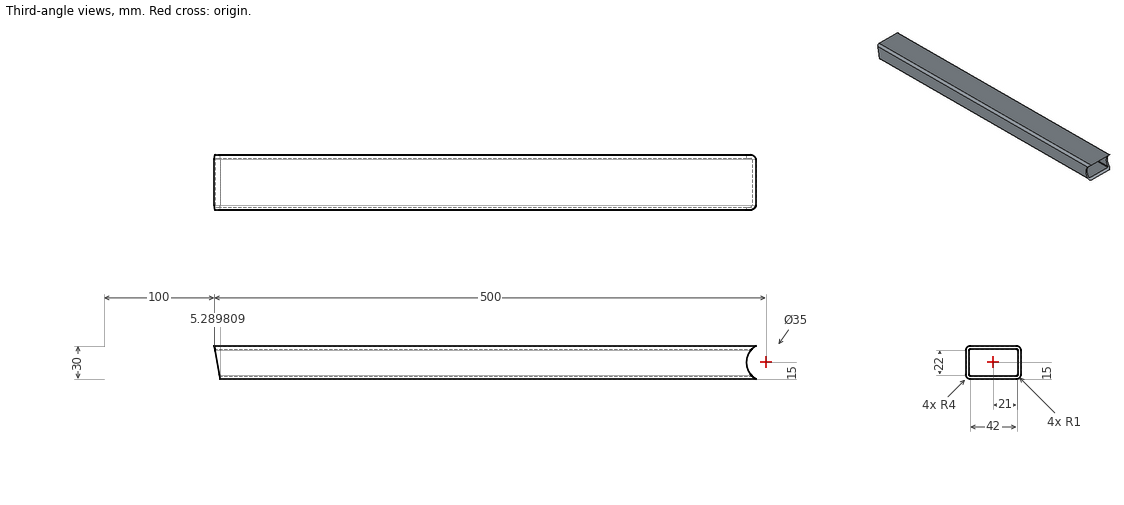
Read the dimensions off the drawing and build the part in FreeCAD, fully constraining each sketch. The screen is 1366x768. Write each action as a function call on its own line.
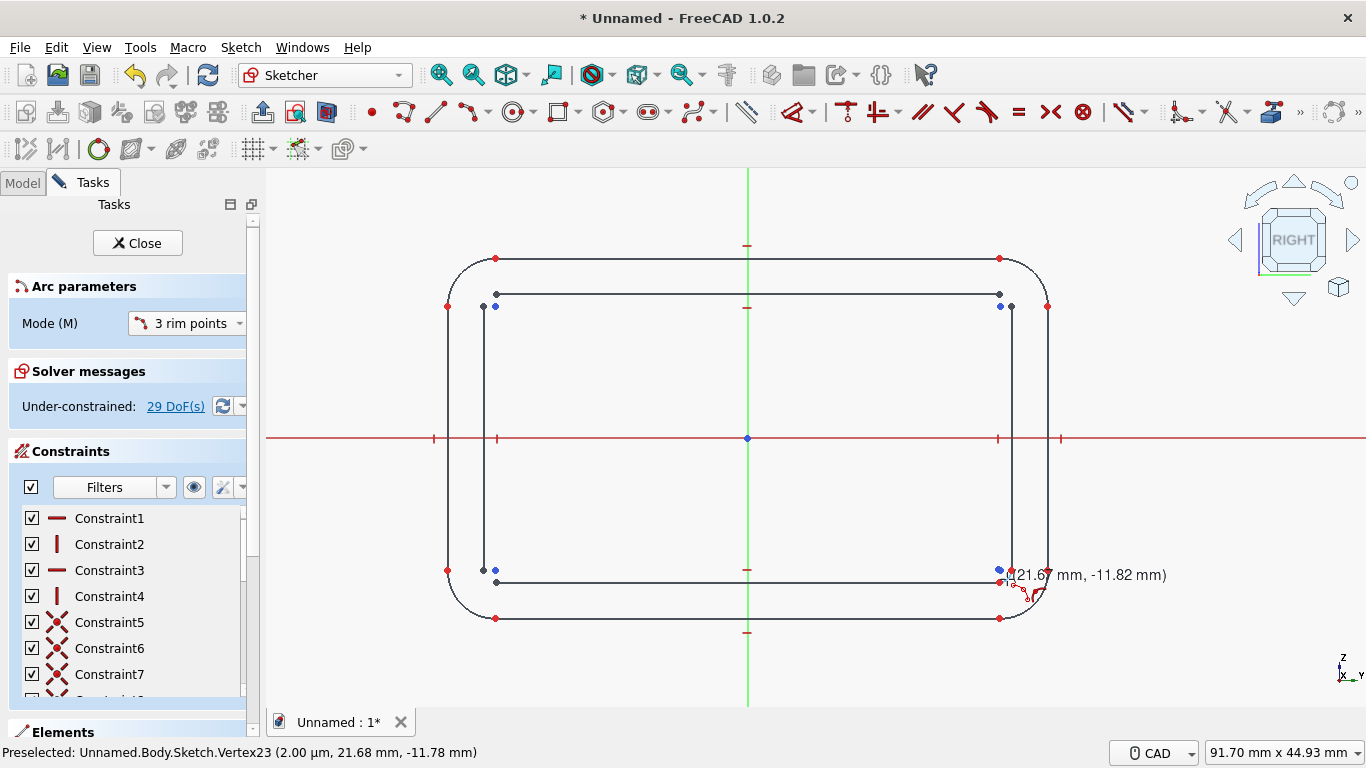
scroll(1012, 306, up, 2)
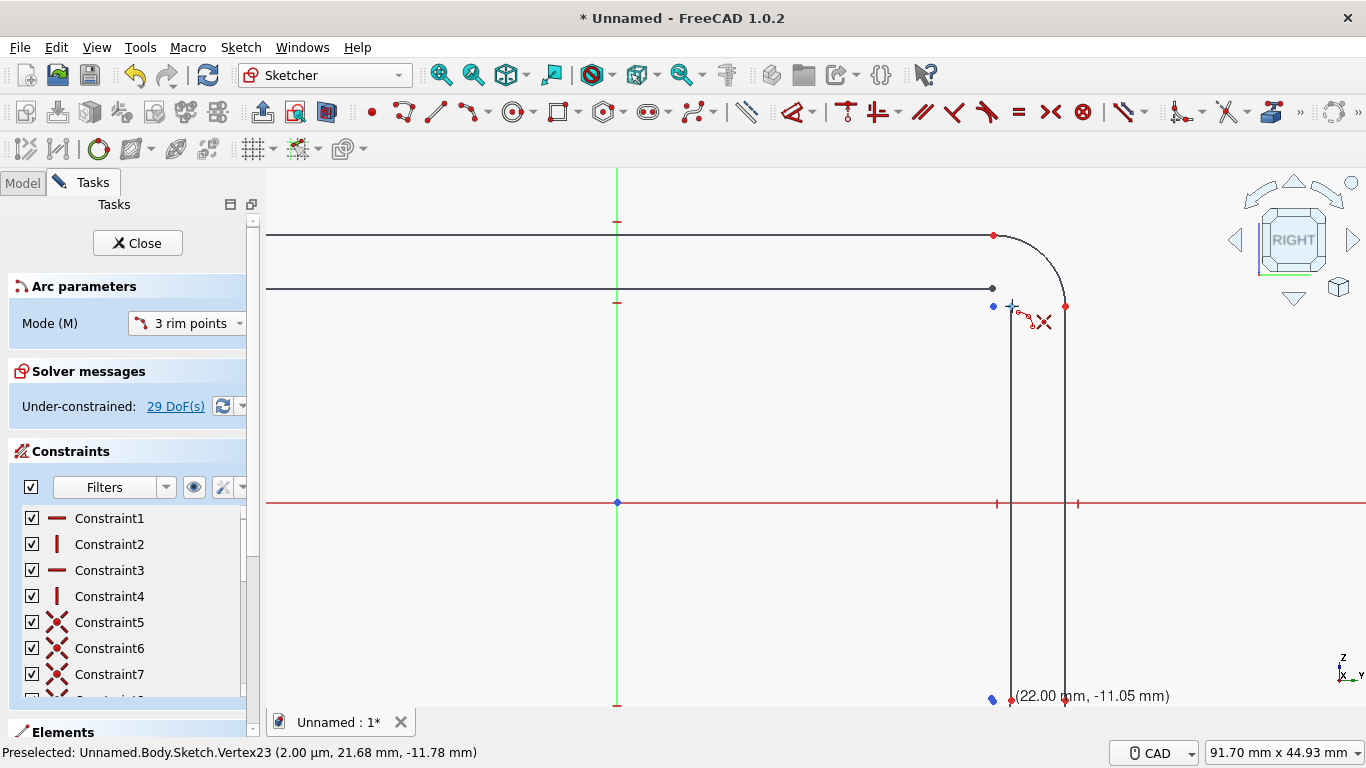
click(1011, 307)
click(993, 289)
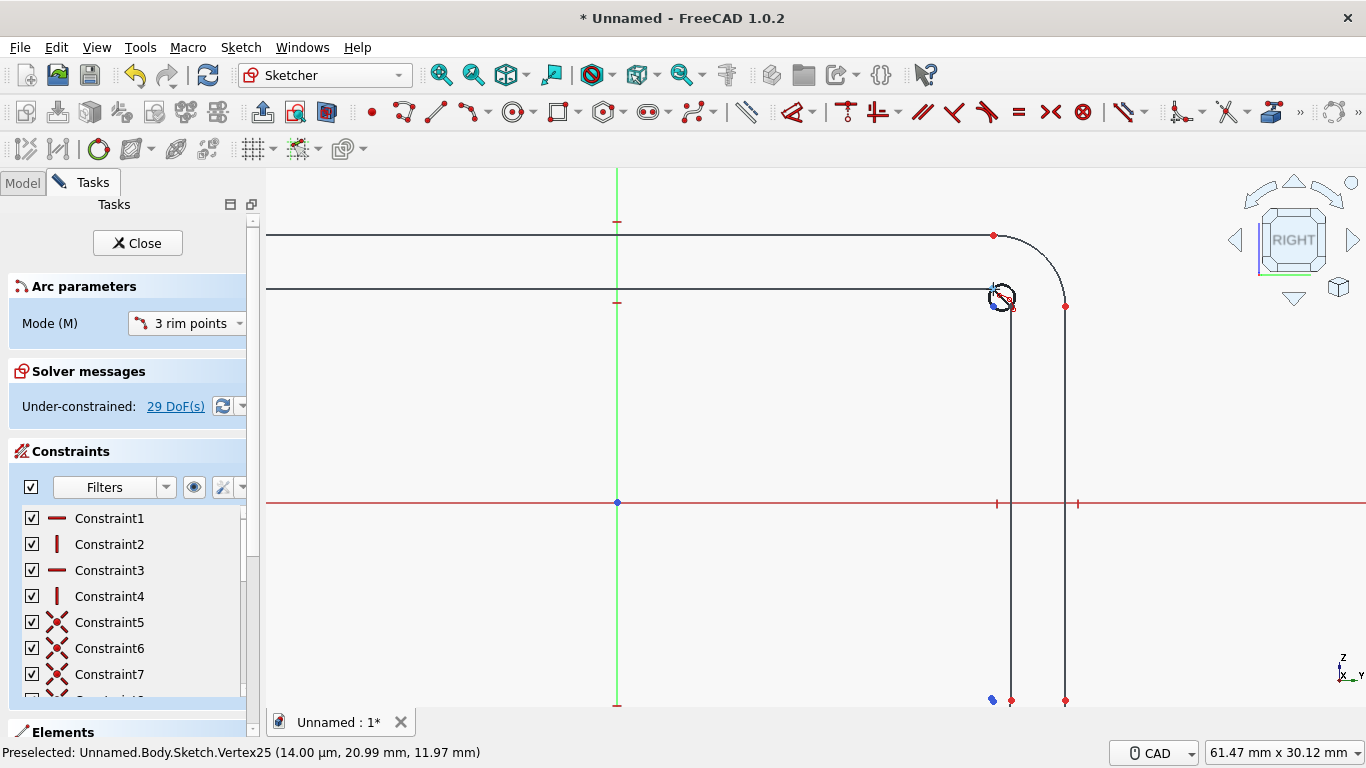
scroll(1006, 293, up, 6)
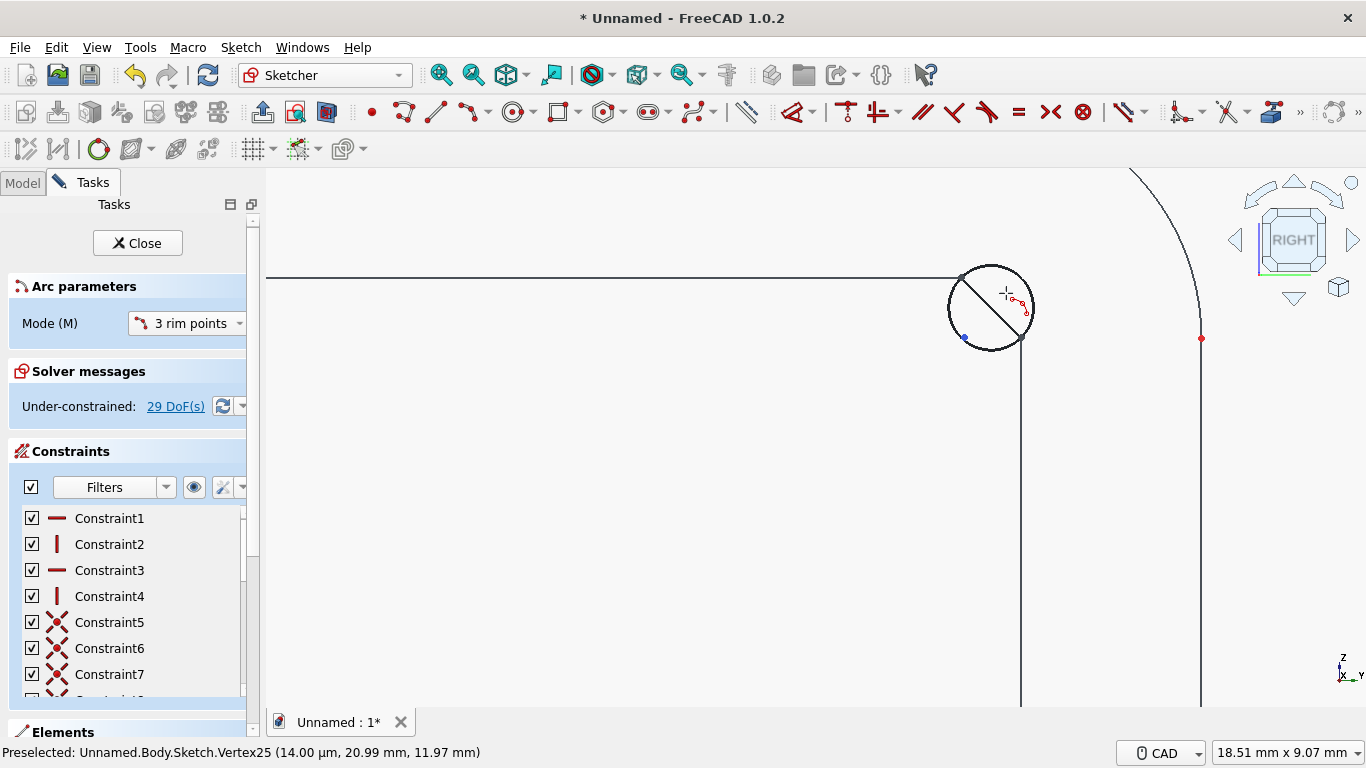
click(1004, 293)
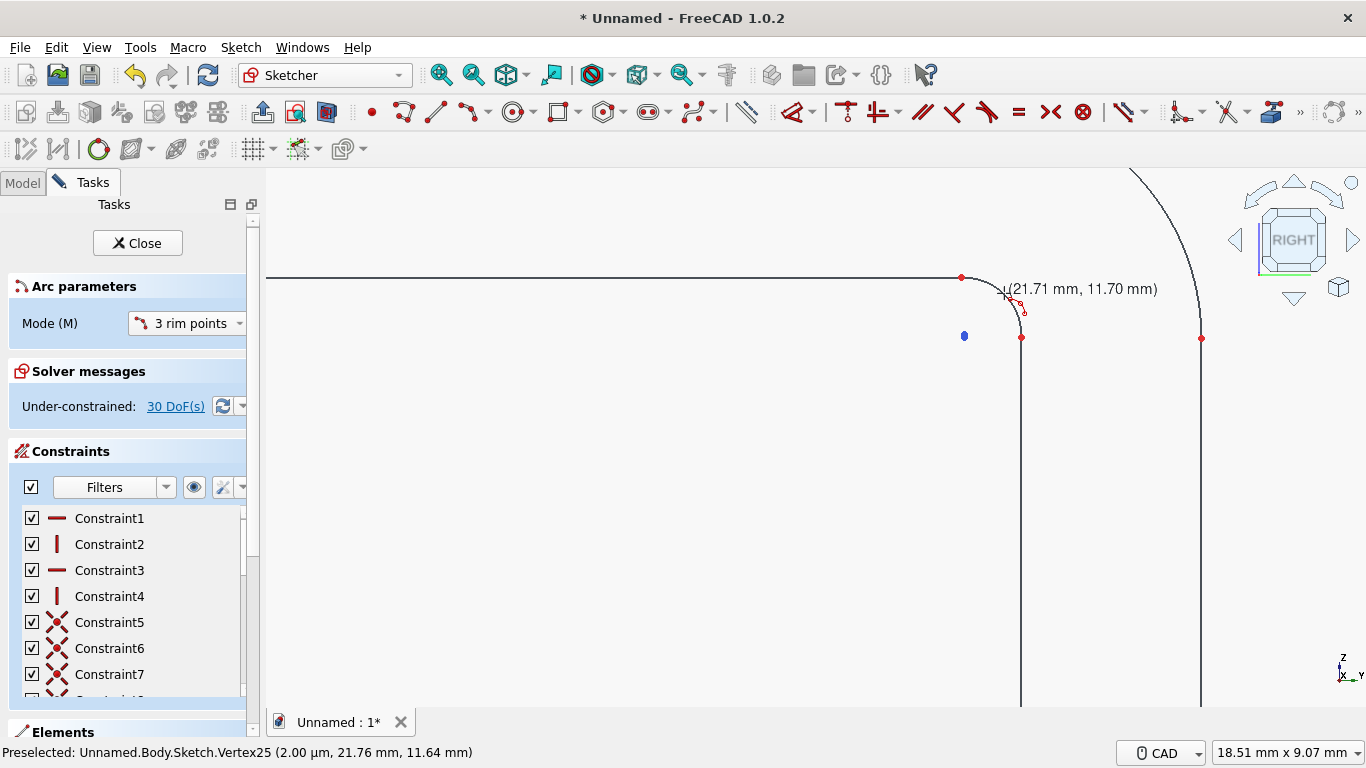
scroll(1009, 298, down, 8)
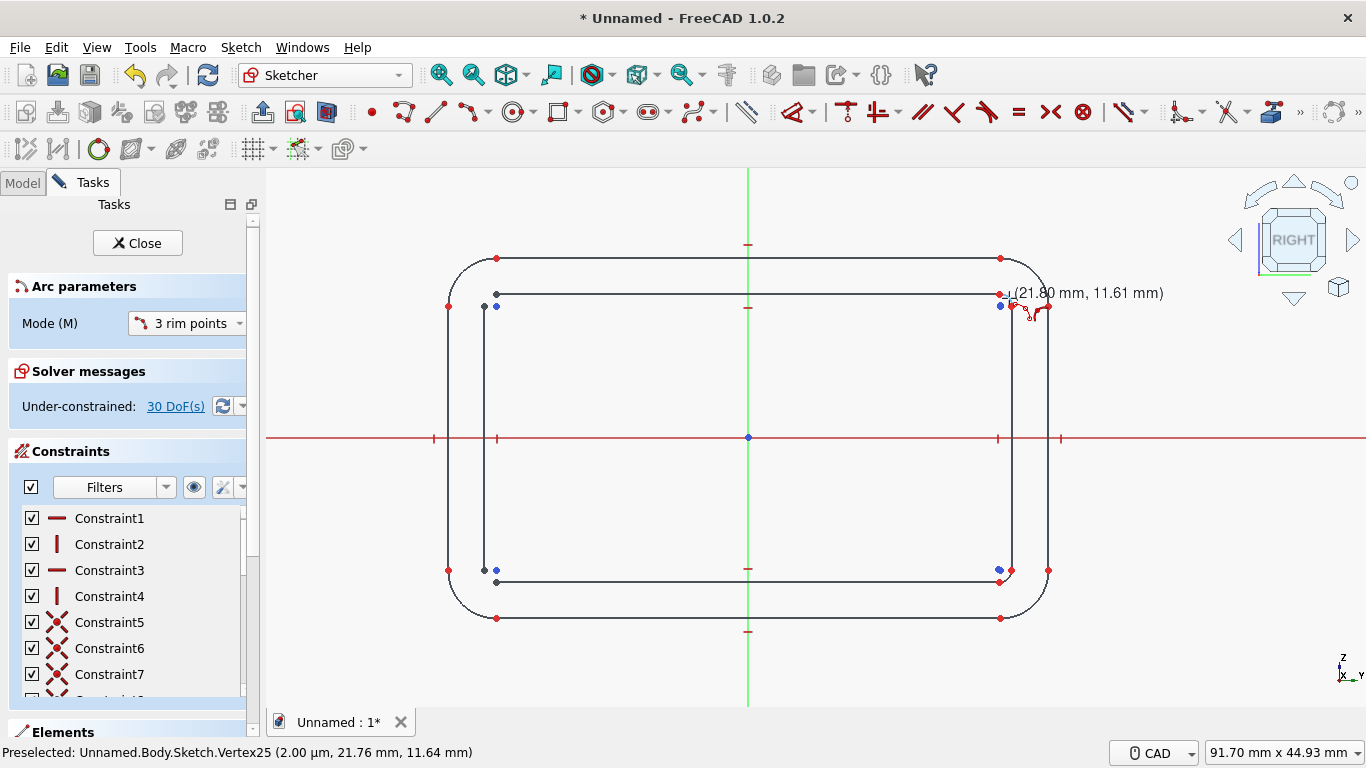
scroll(496, 294, up, 2)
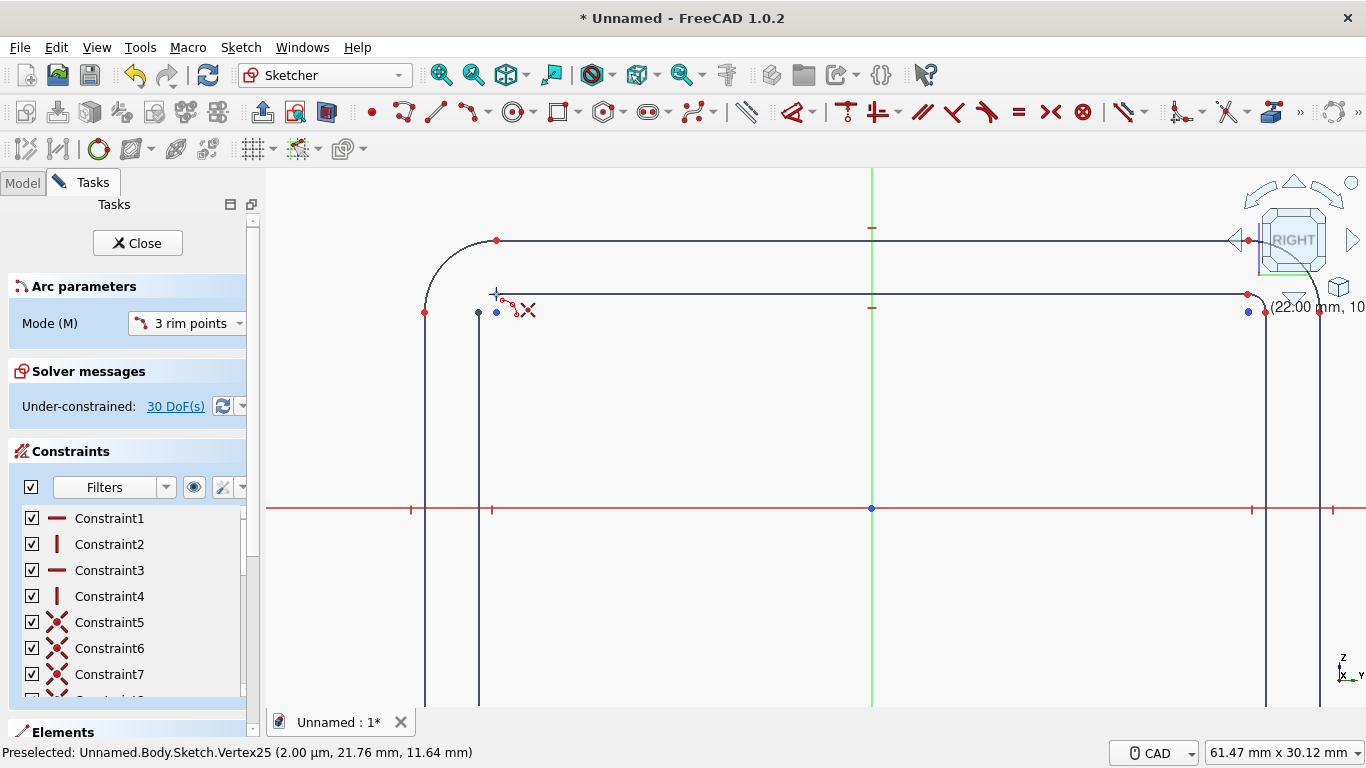
click(497, 294)
click(479, 312)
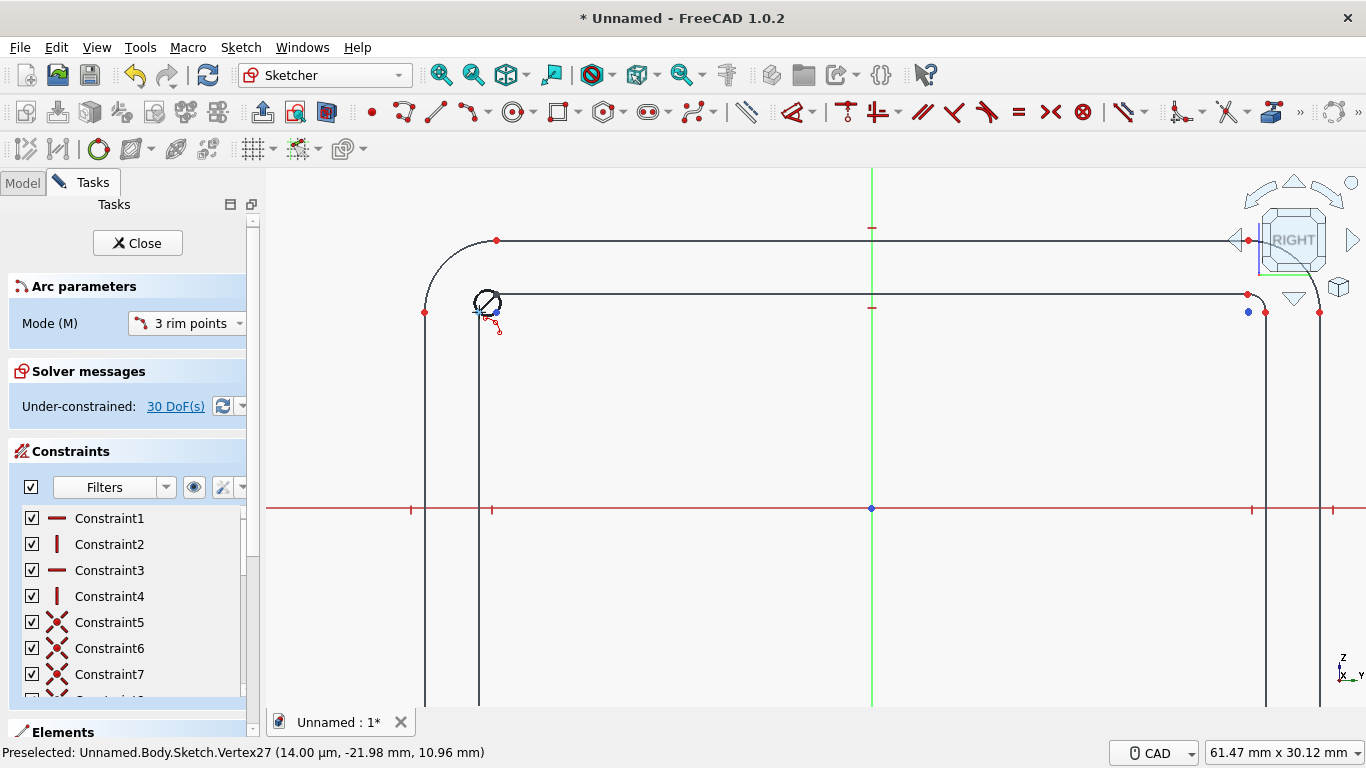
scroll(483, 299, up, 6)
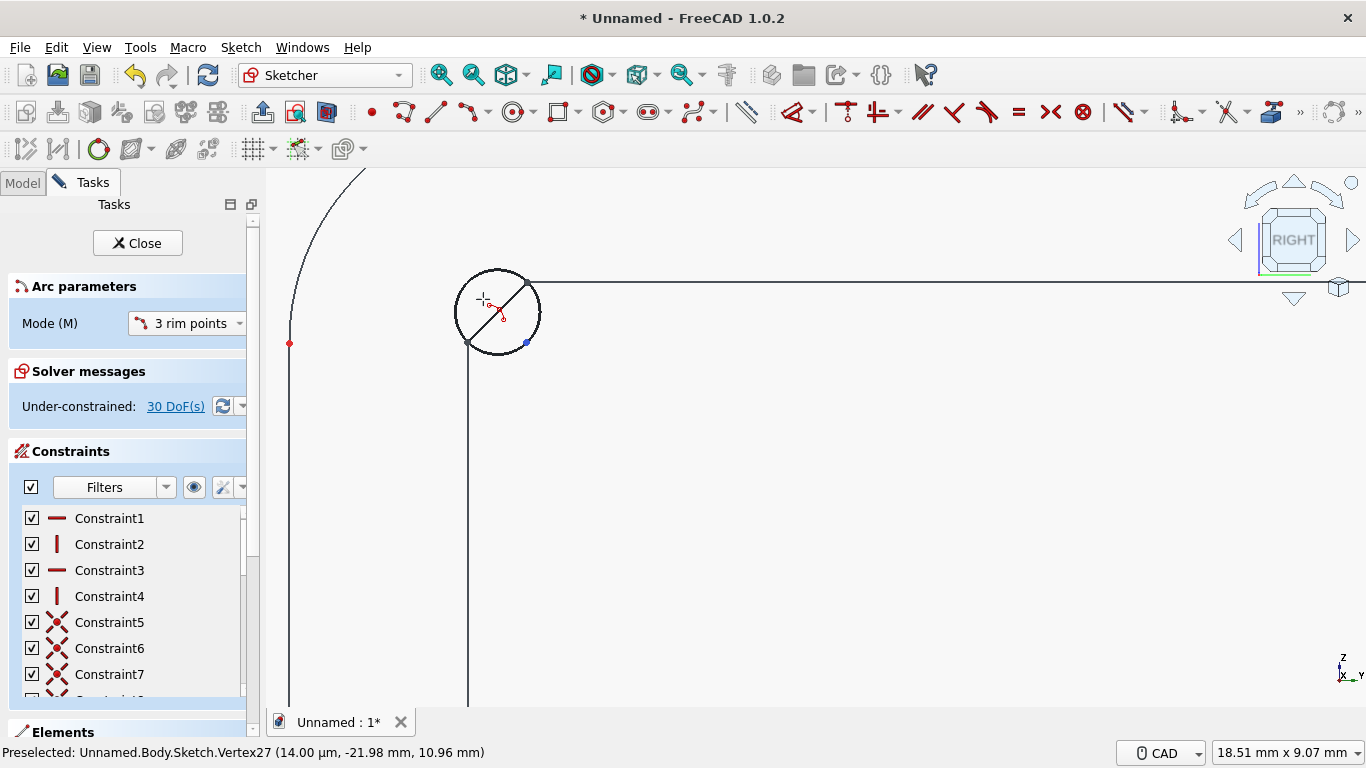
click(484, 298)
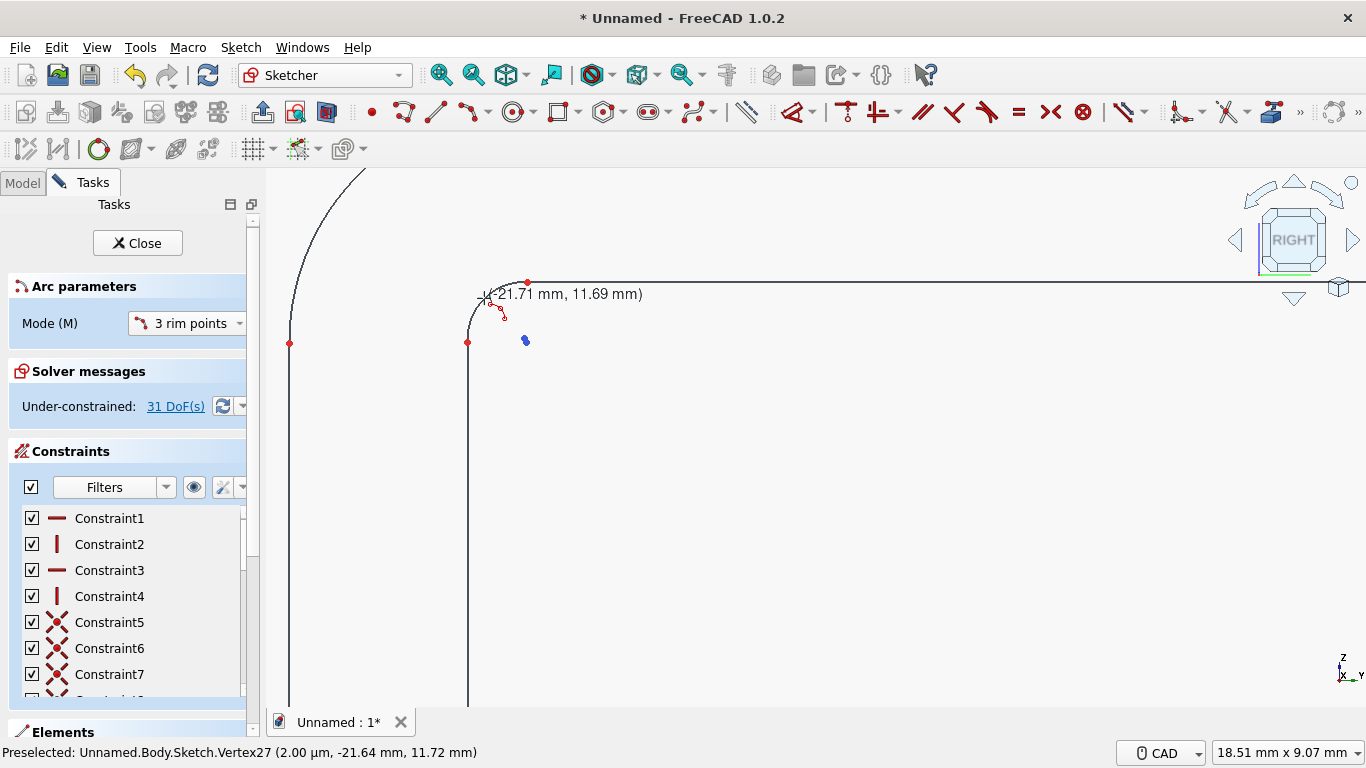
scroll(488, 297, down, 8)